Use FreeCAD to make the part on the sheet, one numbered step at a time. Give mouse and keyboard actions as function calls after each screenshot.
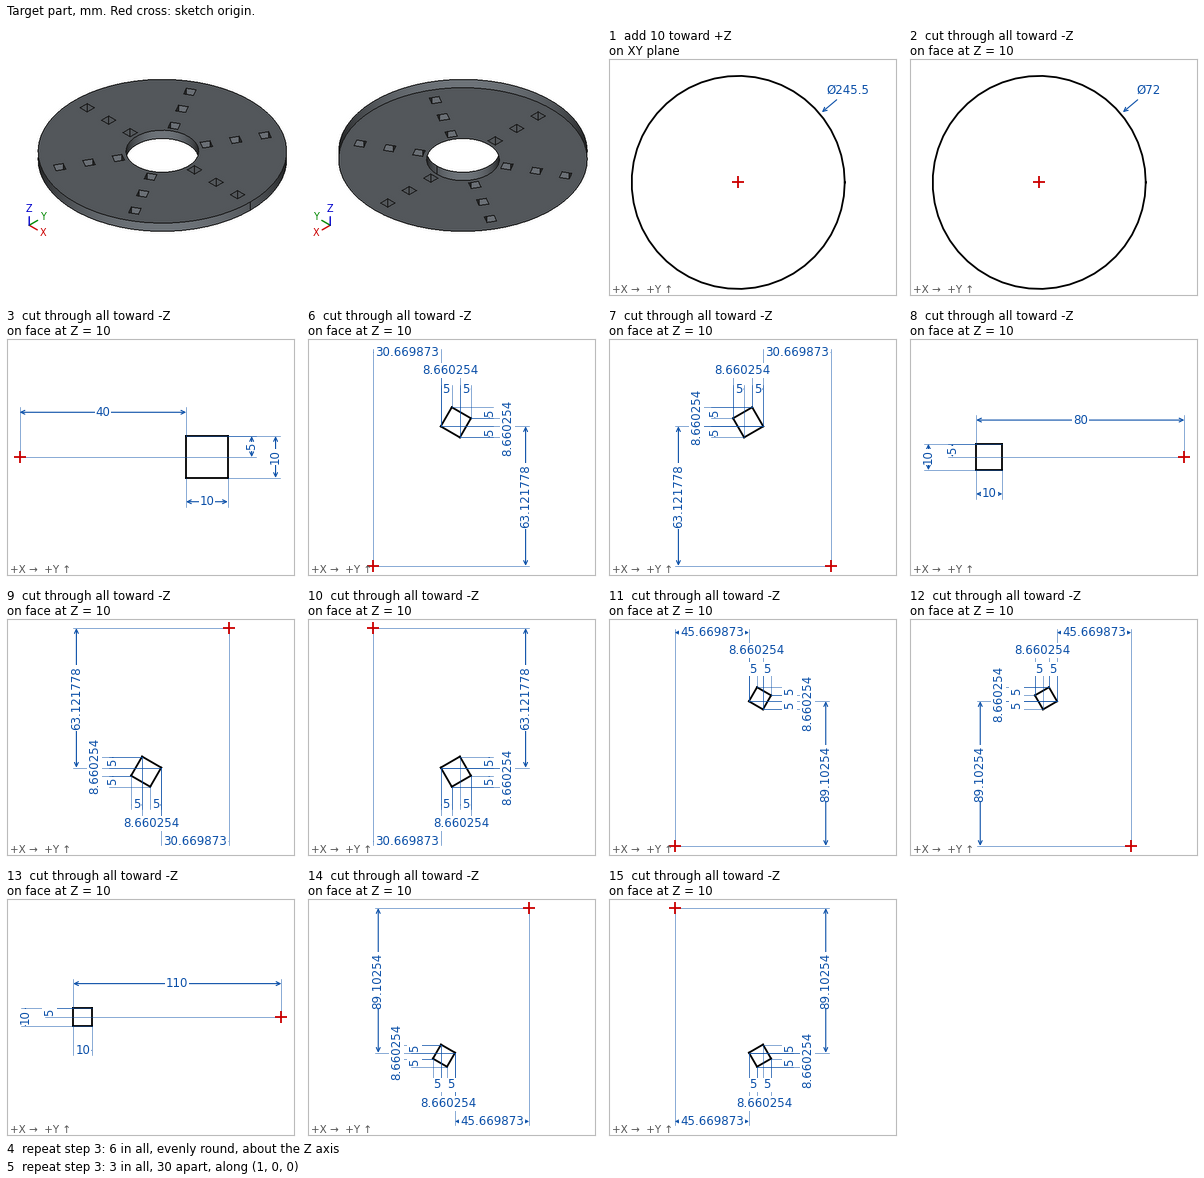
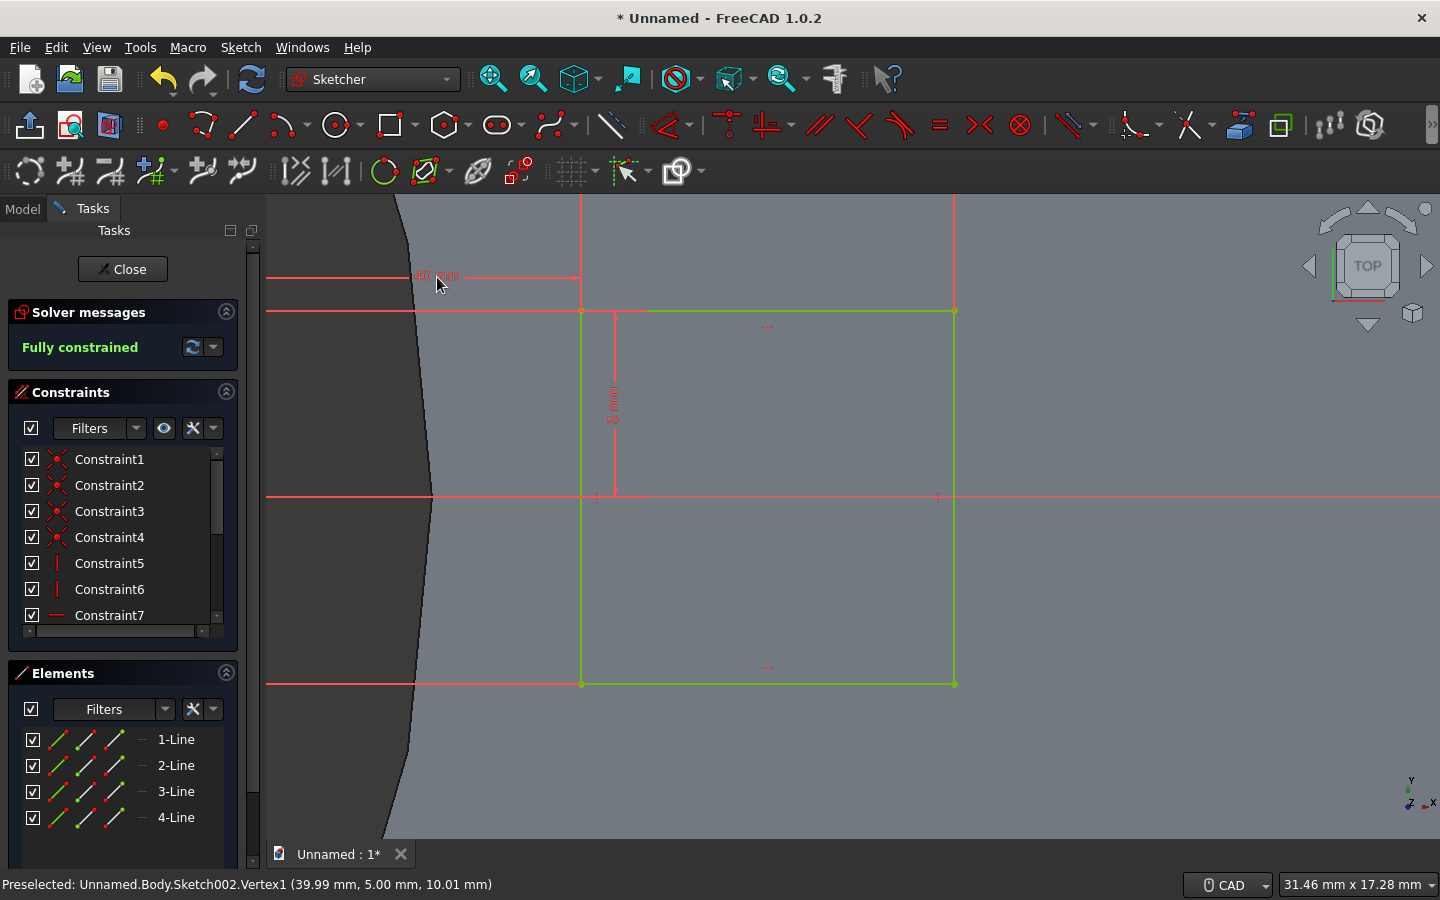
click(123, 269)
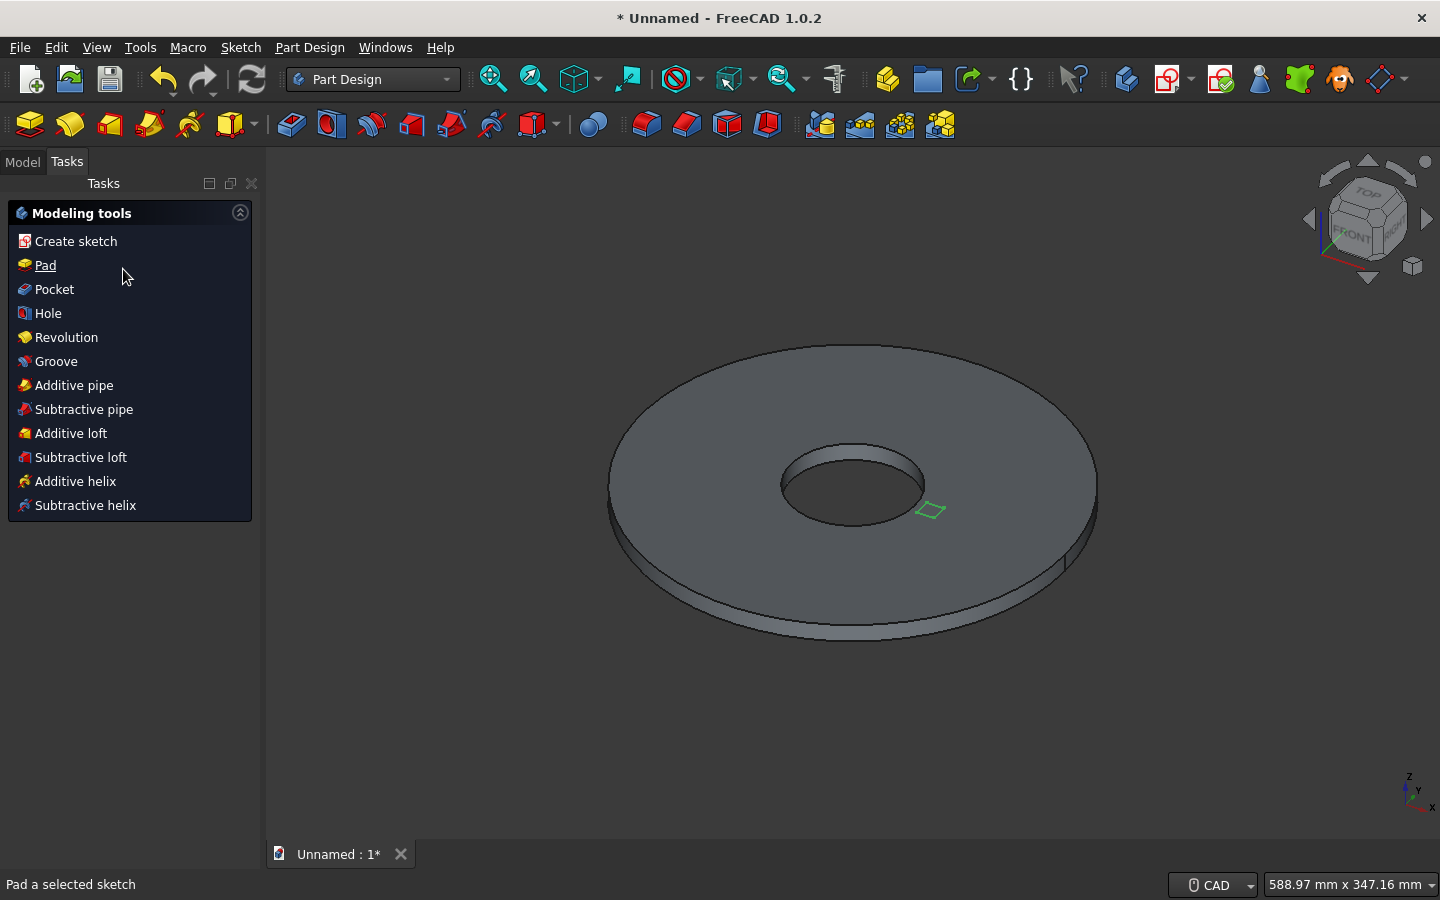
click(292, 124)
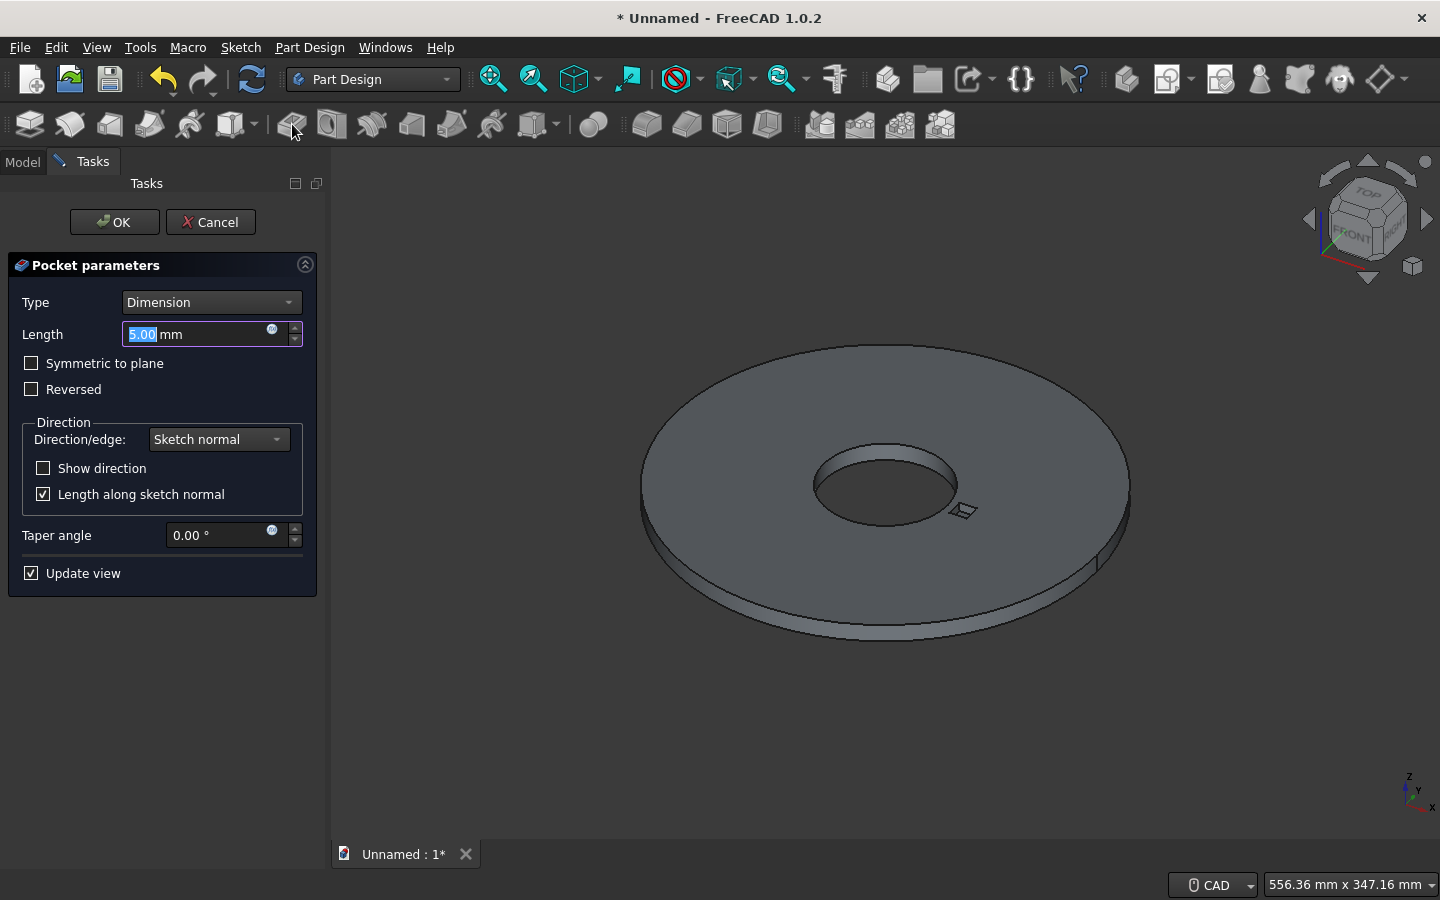
click(212, 302)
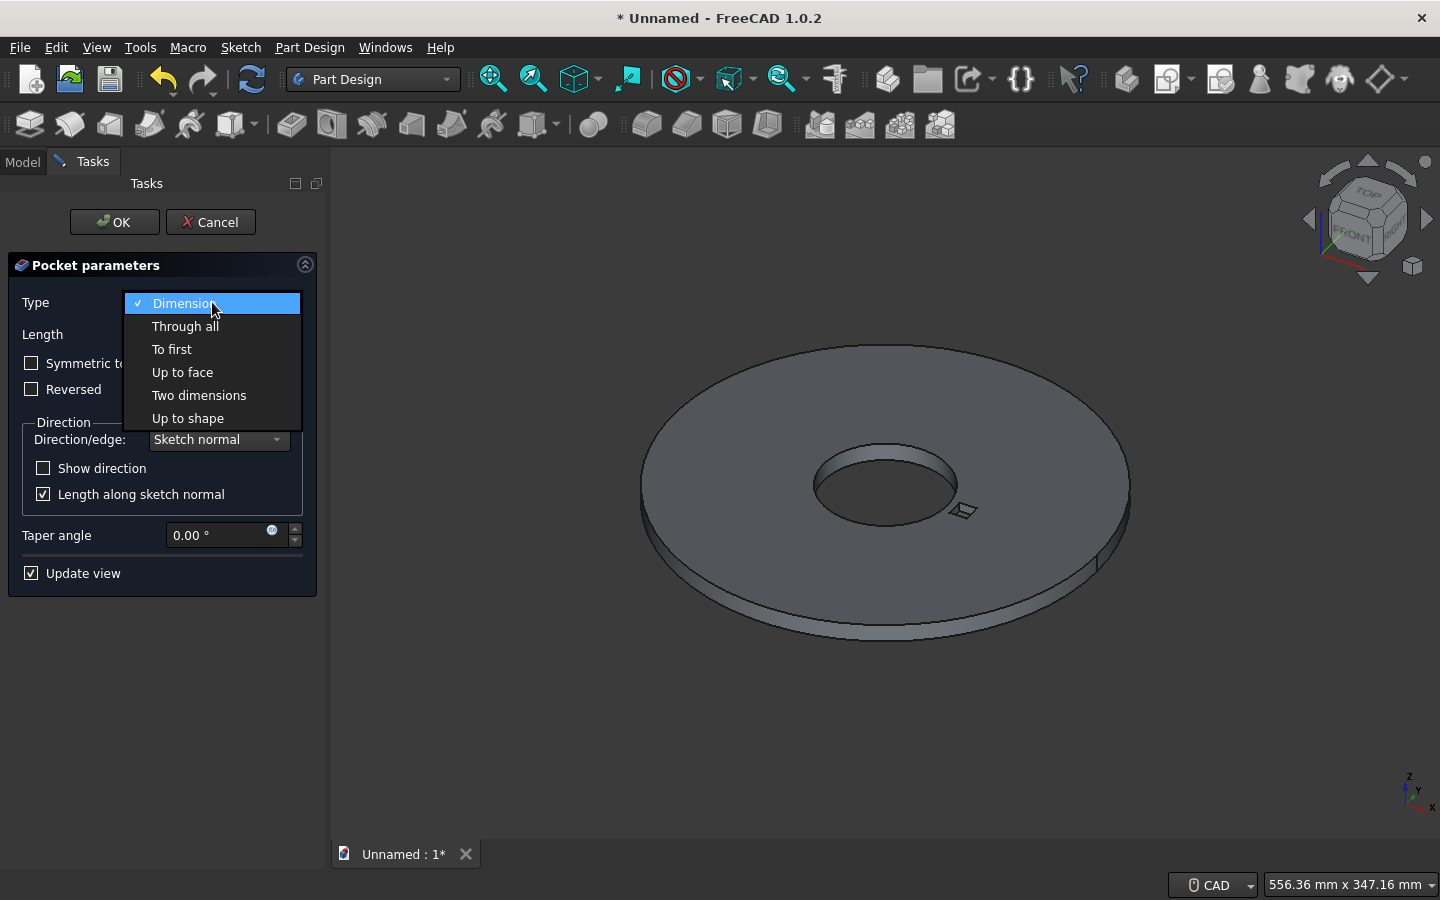
click(212, 326)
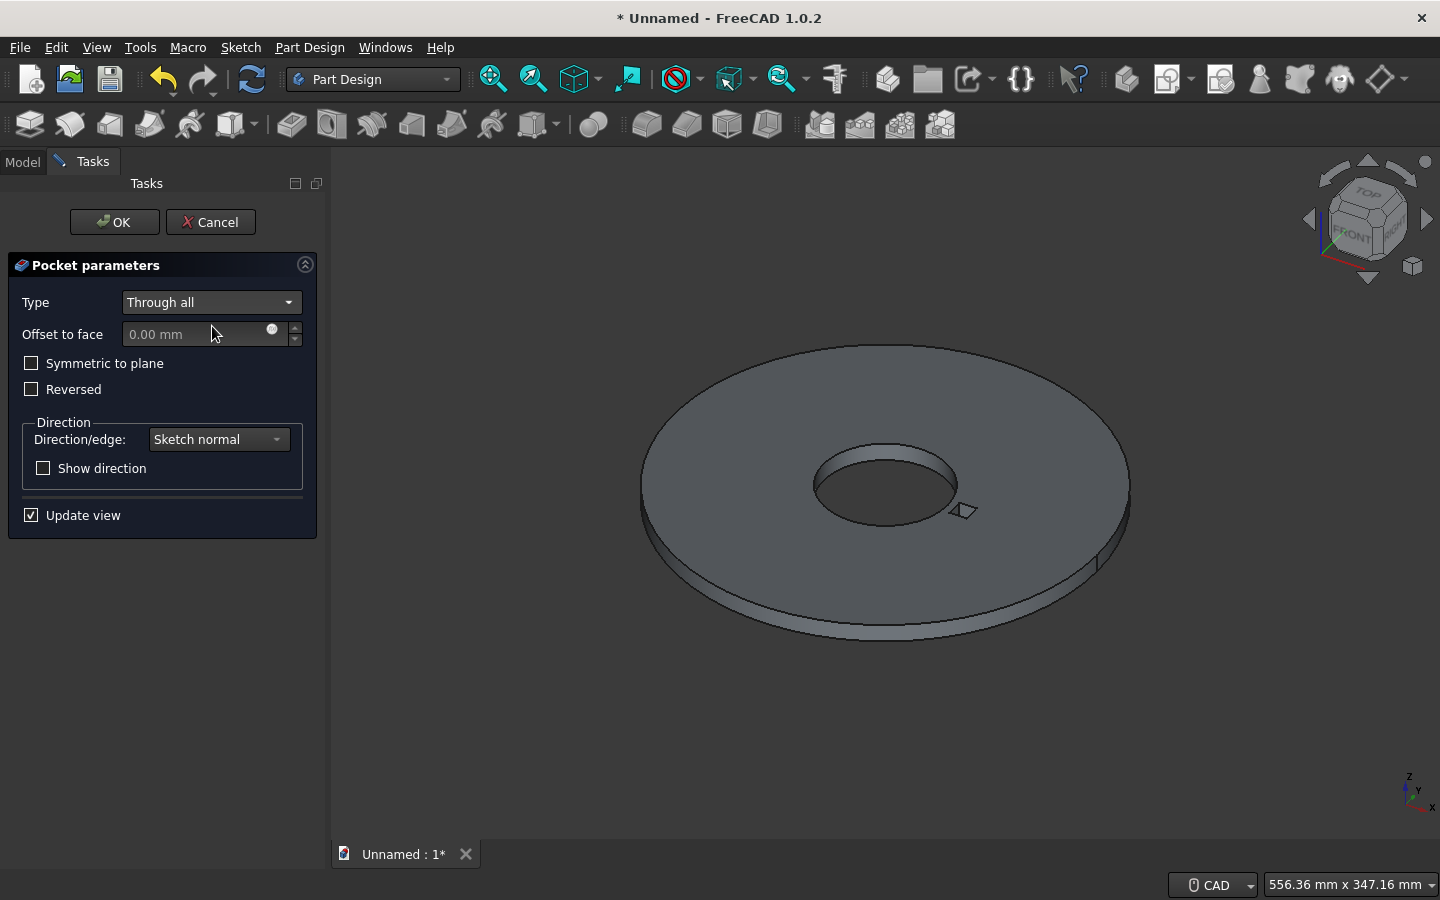
click(115, 222)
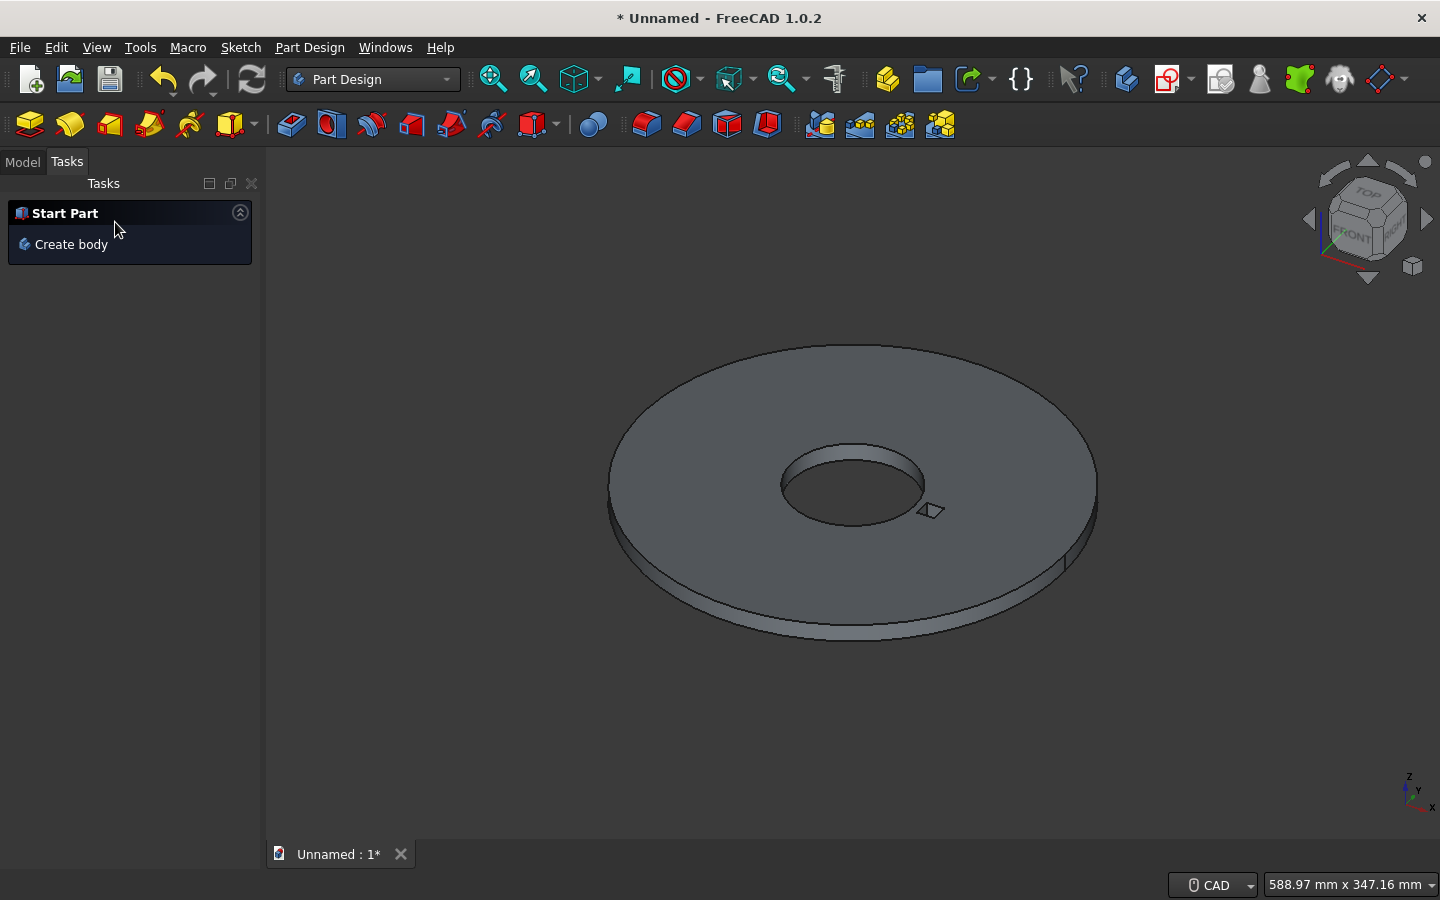
click(23, 161)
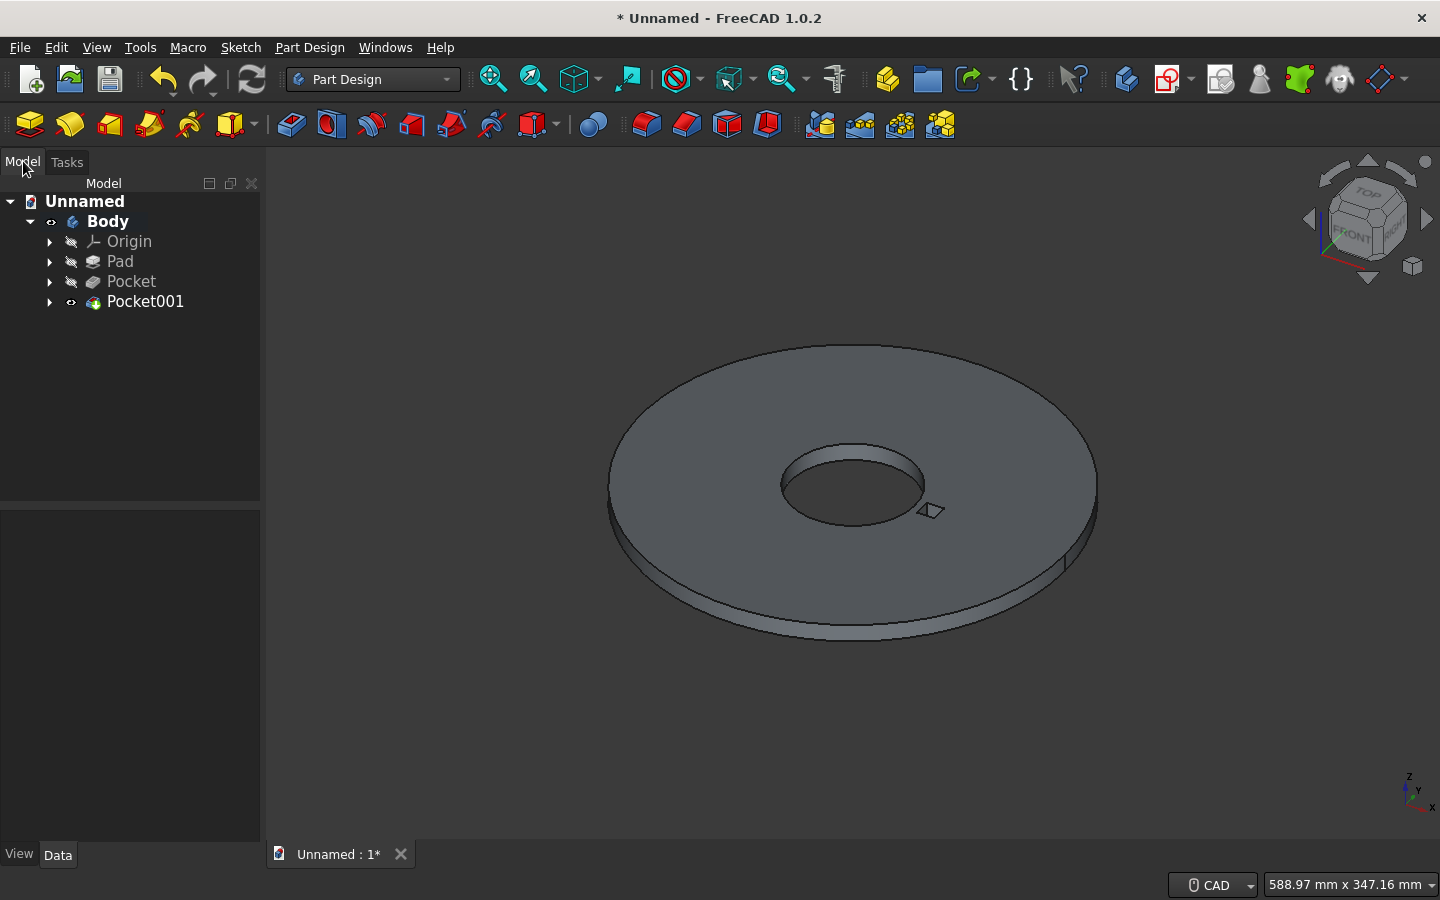
click(116, 302)